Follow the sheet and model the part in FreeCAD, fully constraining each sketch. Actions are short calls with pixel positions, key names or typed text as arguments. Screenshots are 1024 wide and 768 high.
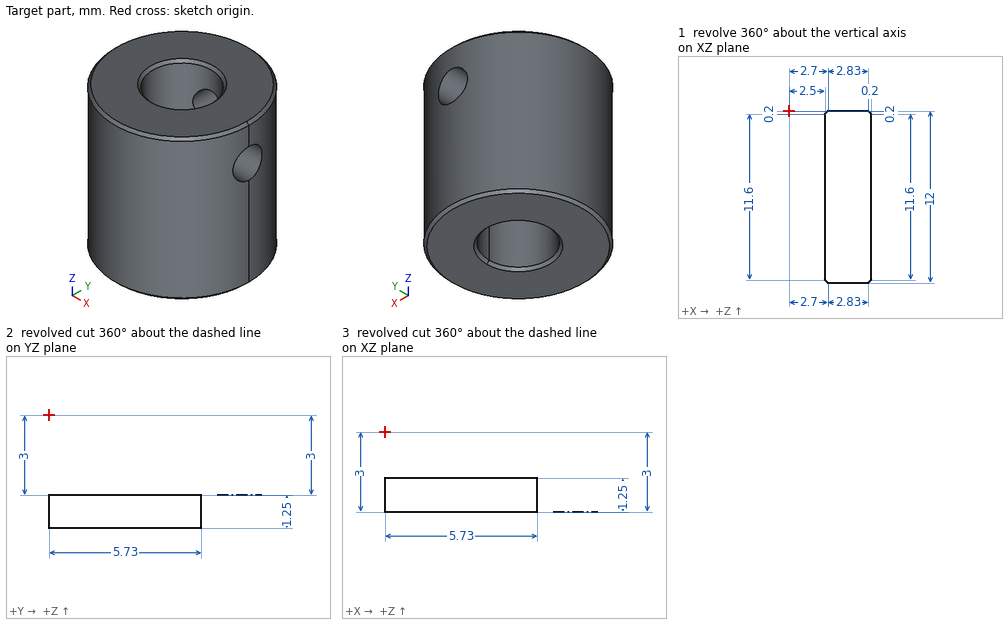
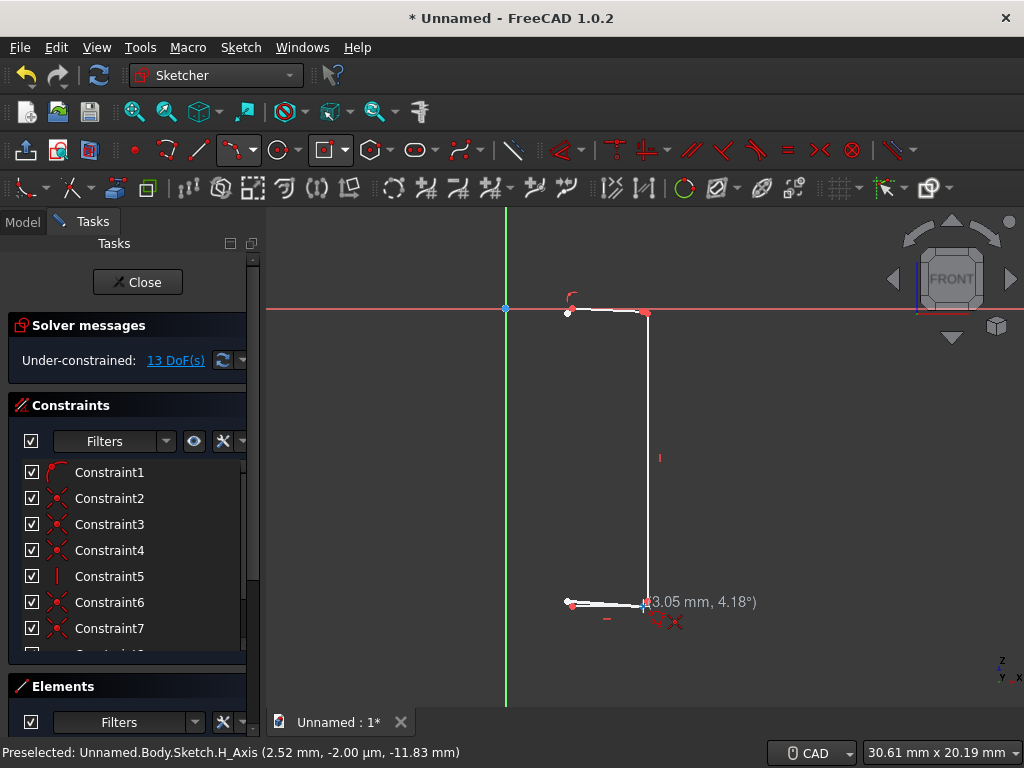
scroll(568, 314, up, 8)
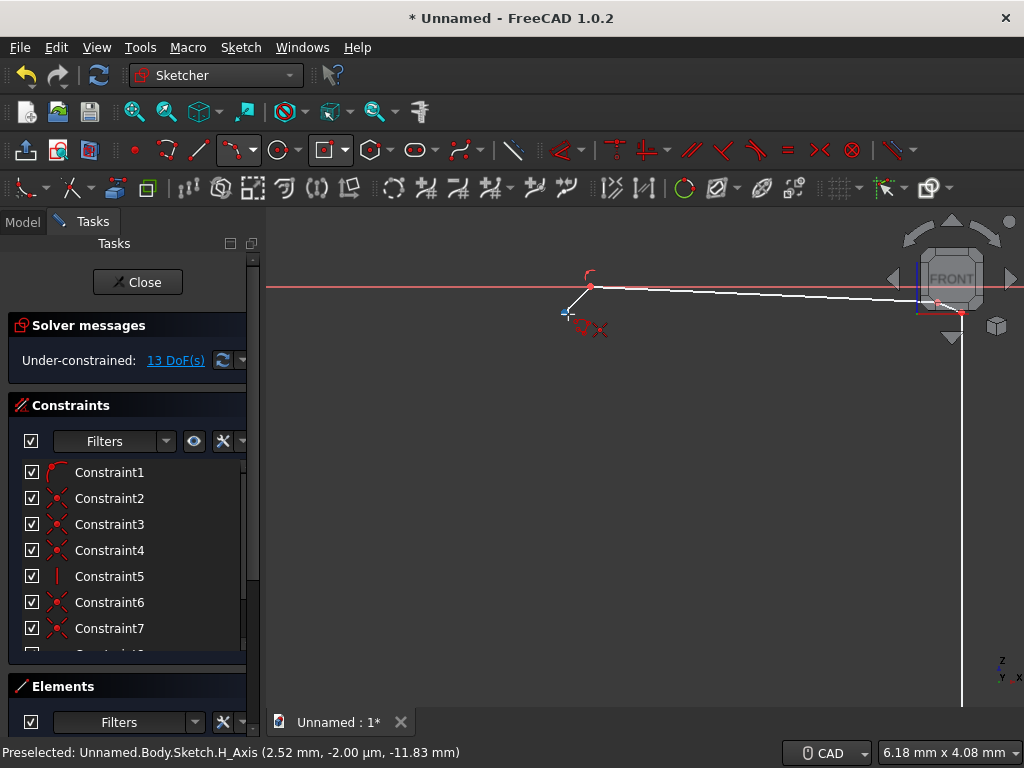
click(565, 313)
key(Escape)
key(Escape)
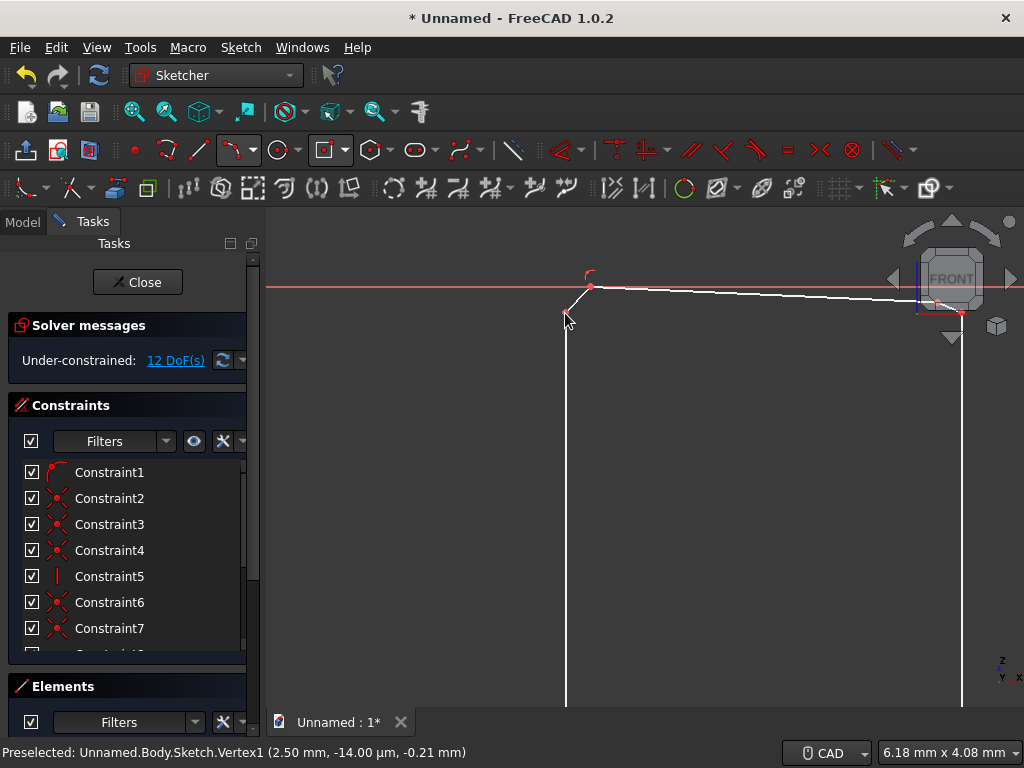
scroll(833, 298, up, 2)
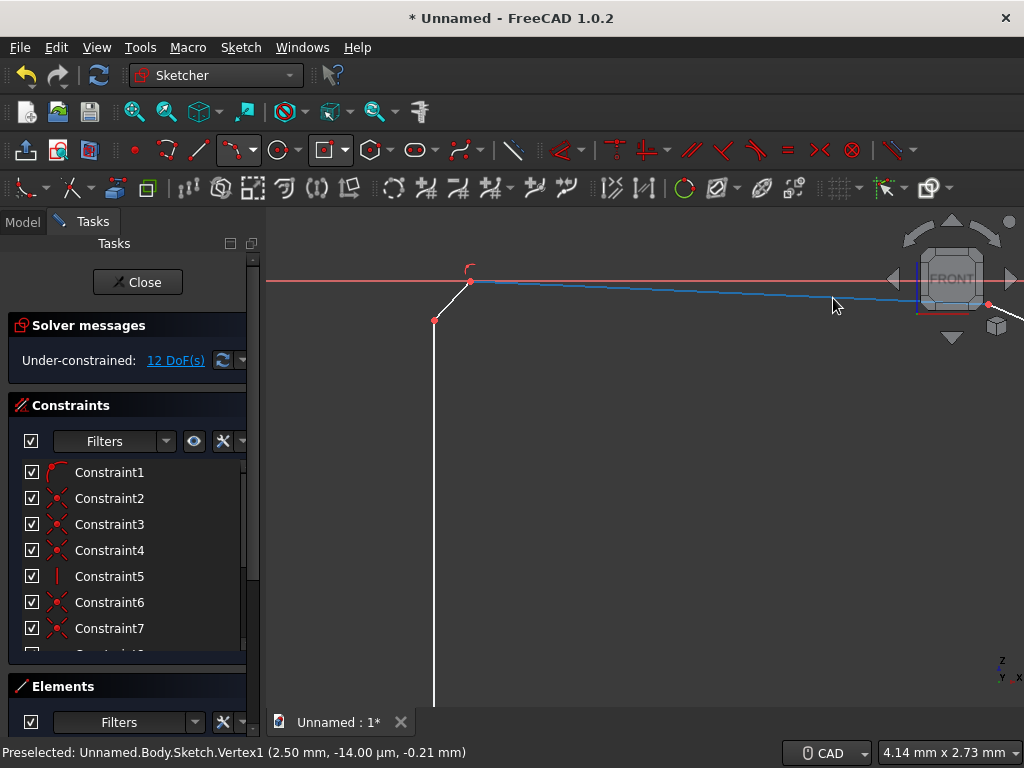
click(833, 298)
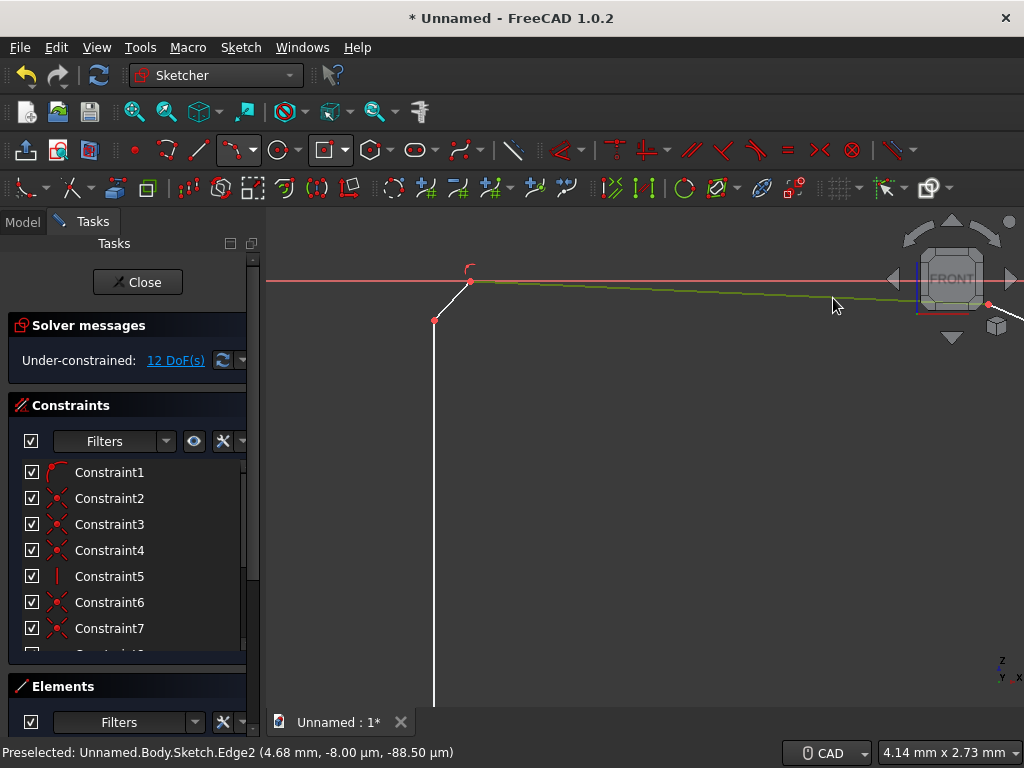
click(670, 150)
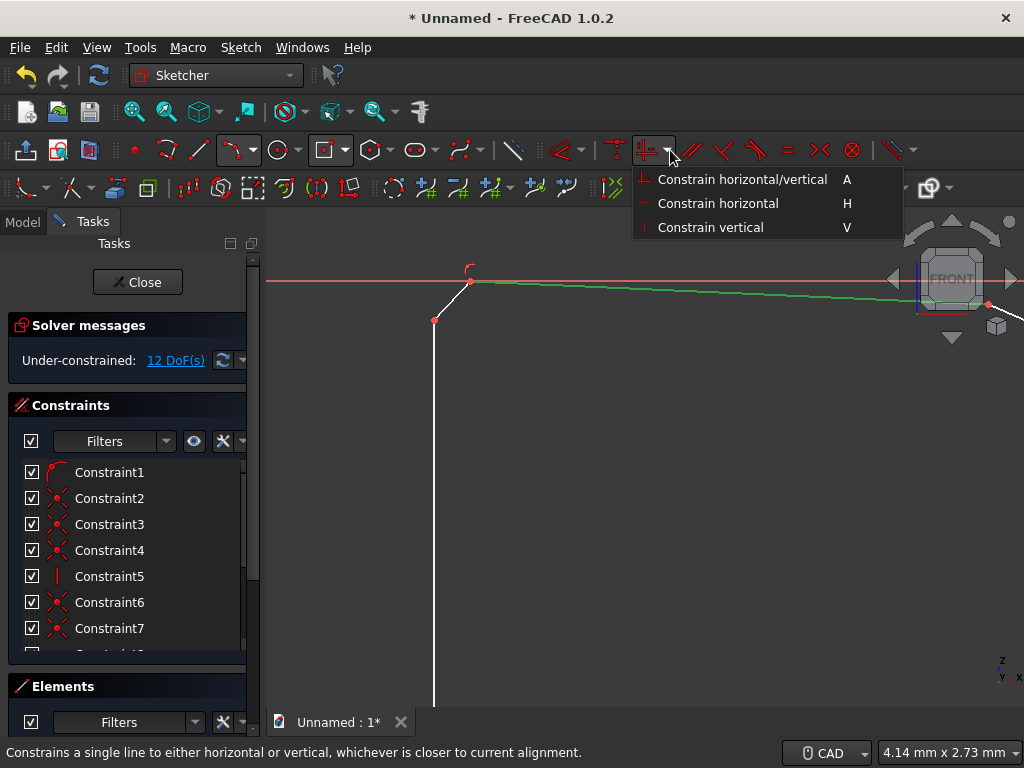
click(768, 203)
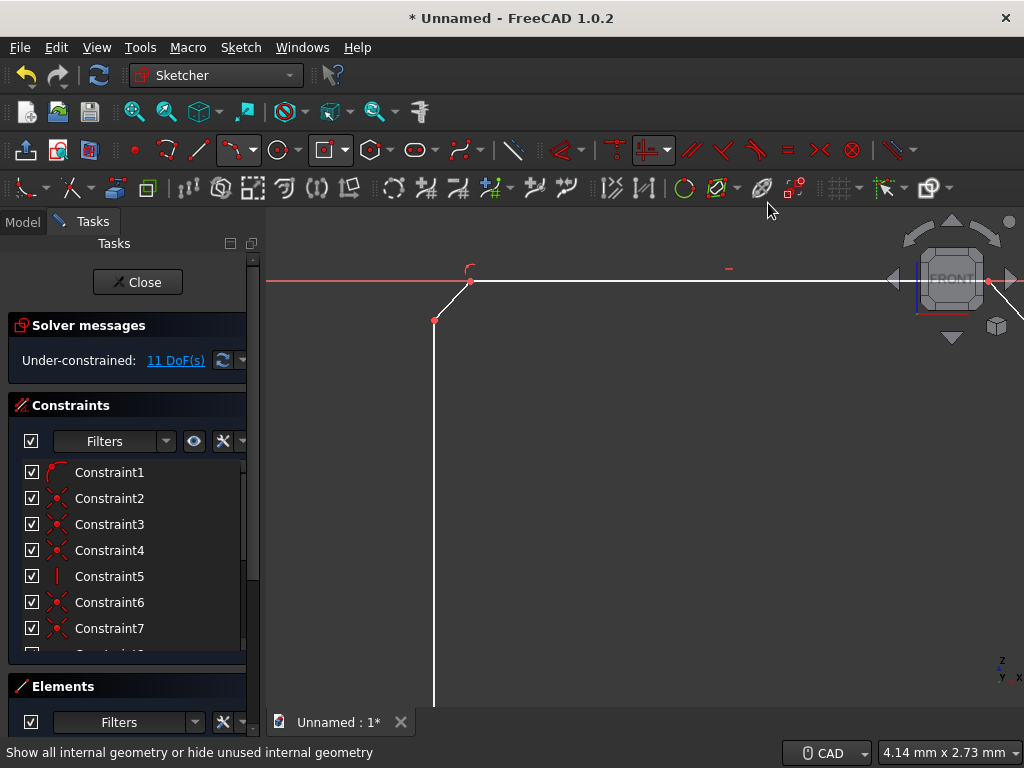
click(560, 150)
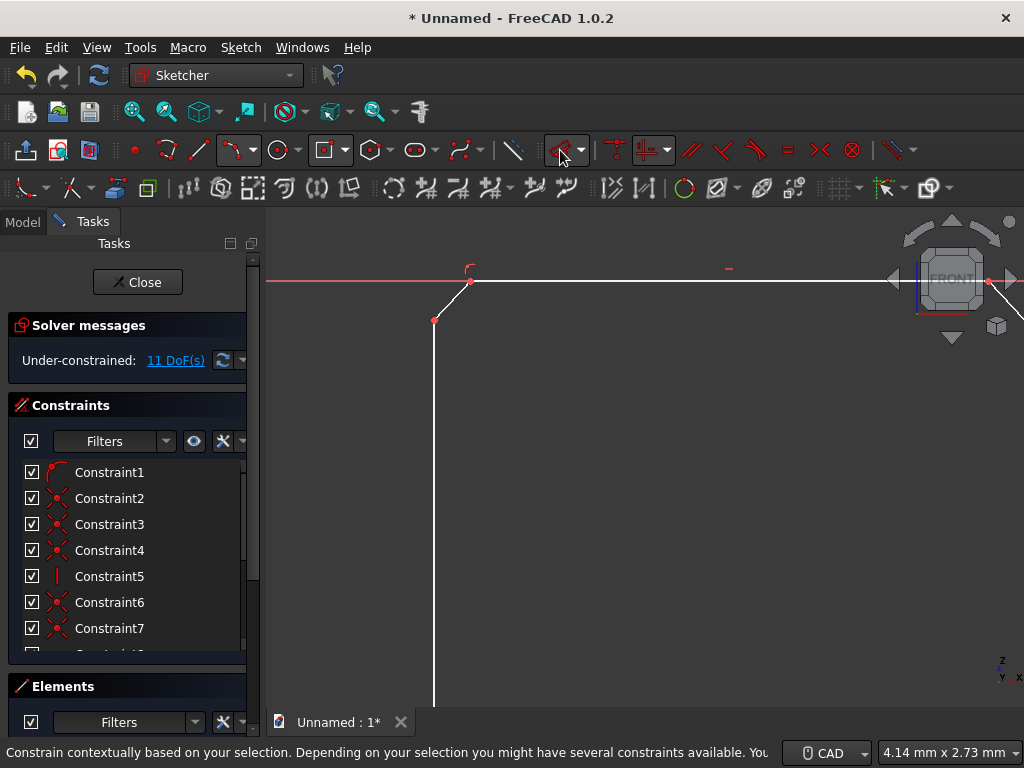
scroll(588, 313, down, 10)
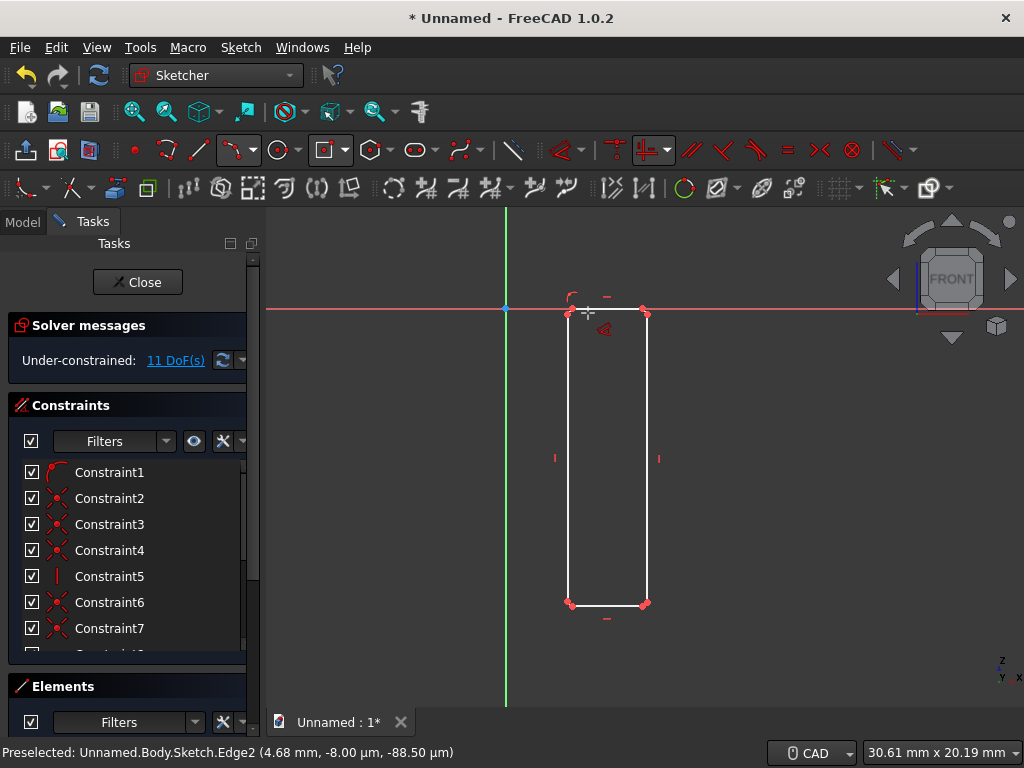
scroll(643, 606, up, 4)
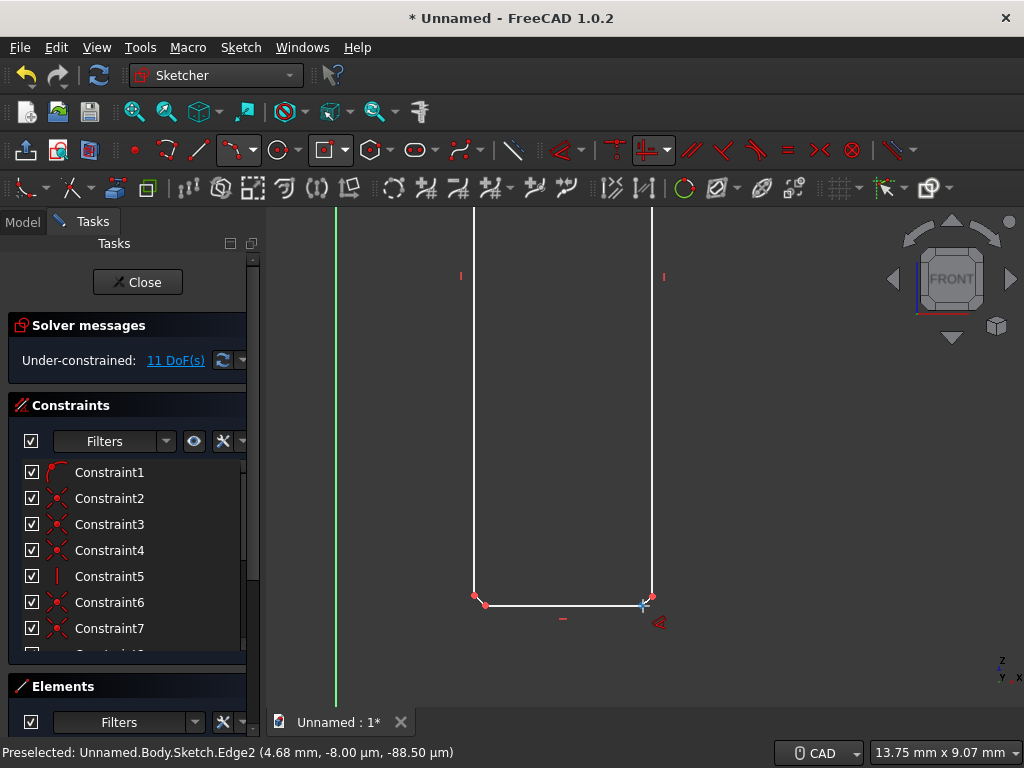
click(642, 606)
click(302, 420)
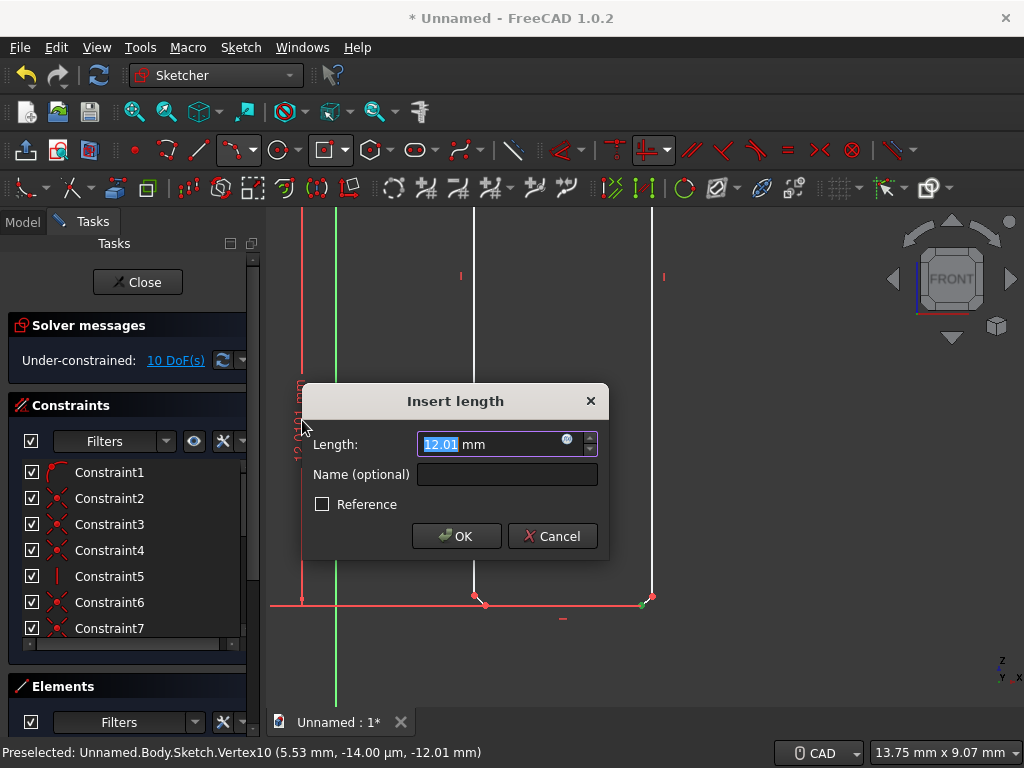
text(12)
key(Return)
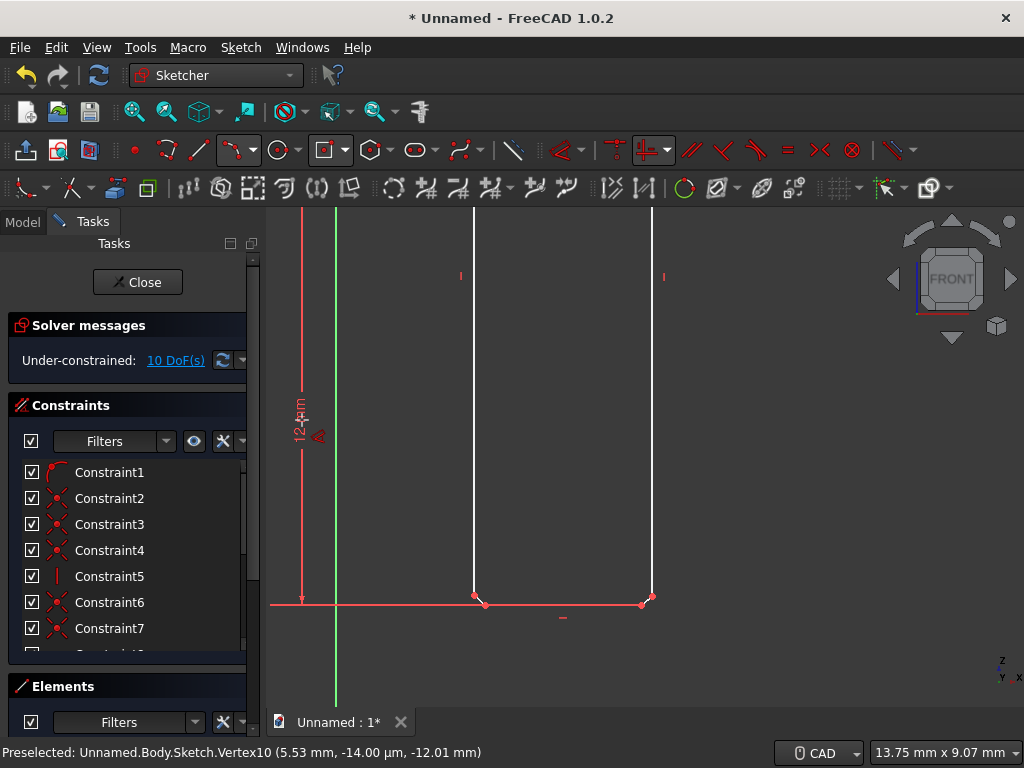
scroll(644, 606, down, 4)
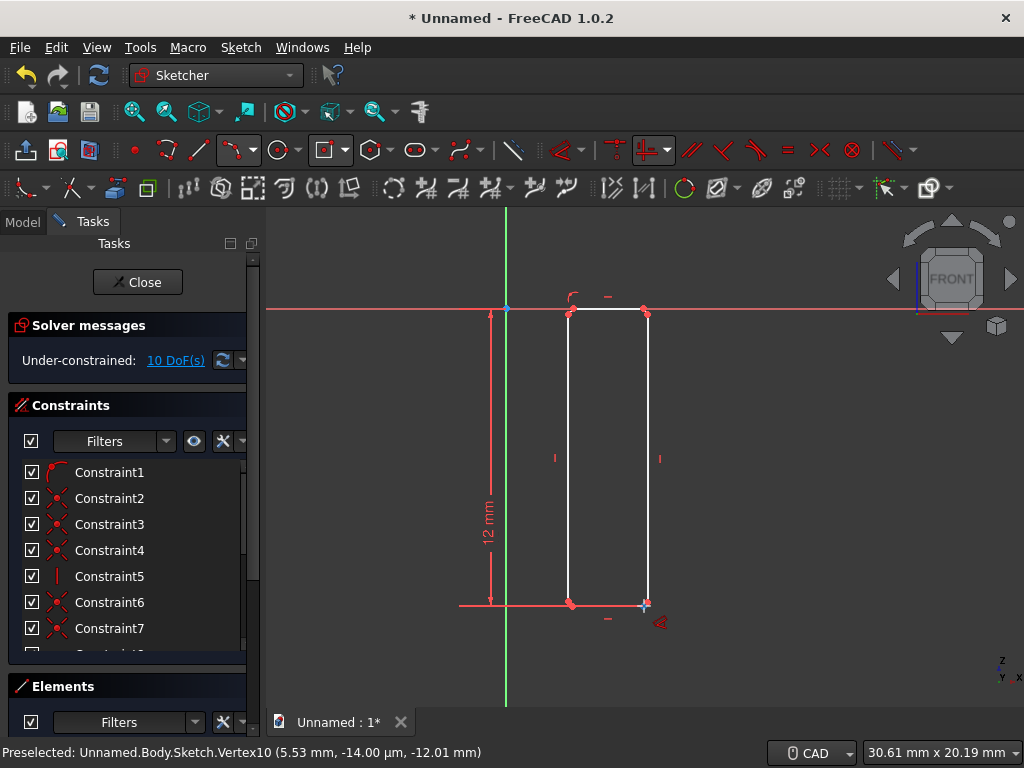
click(594, 309)
click(608, 275)